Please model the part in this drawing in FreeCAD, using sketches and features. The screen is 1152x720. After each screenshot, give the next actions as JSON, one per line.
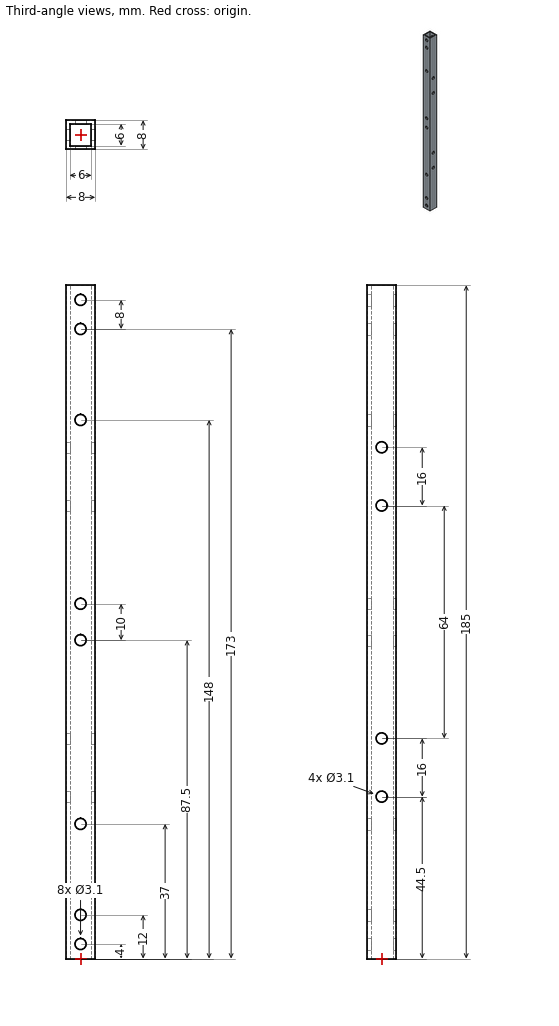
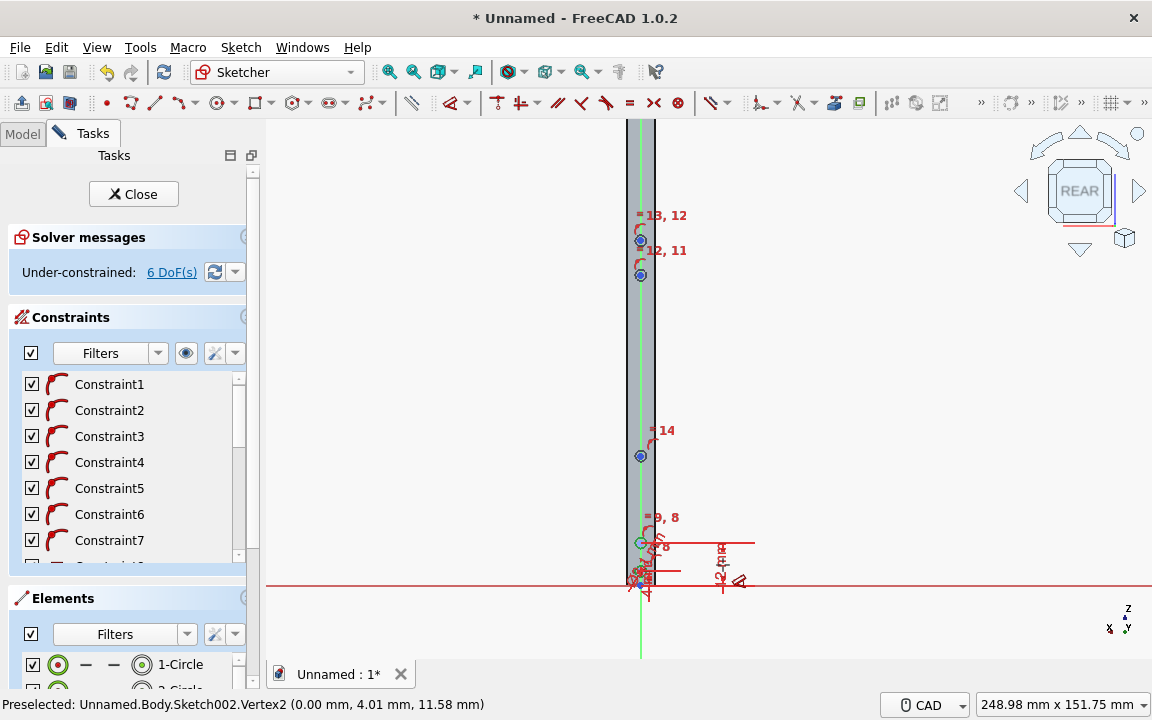
{"action": "left_click", "coordinate": [641, 456]}
{"action": "left_click", "coordinate": [675, 521]}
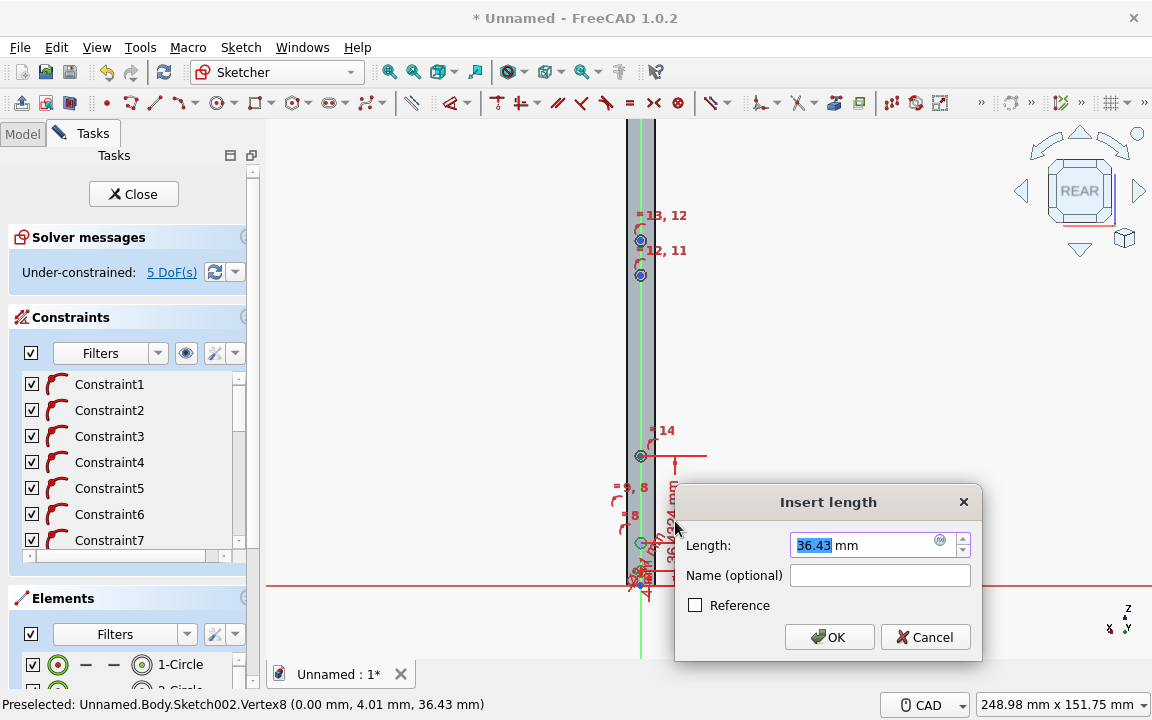
{"action": "type", "text": "37"}
{"action": "key", "text": "Return"}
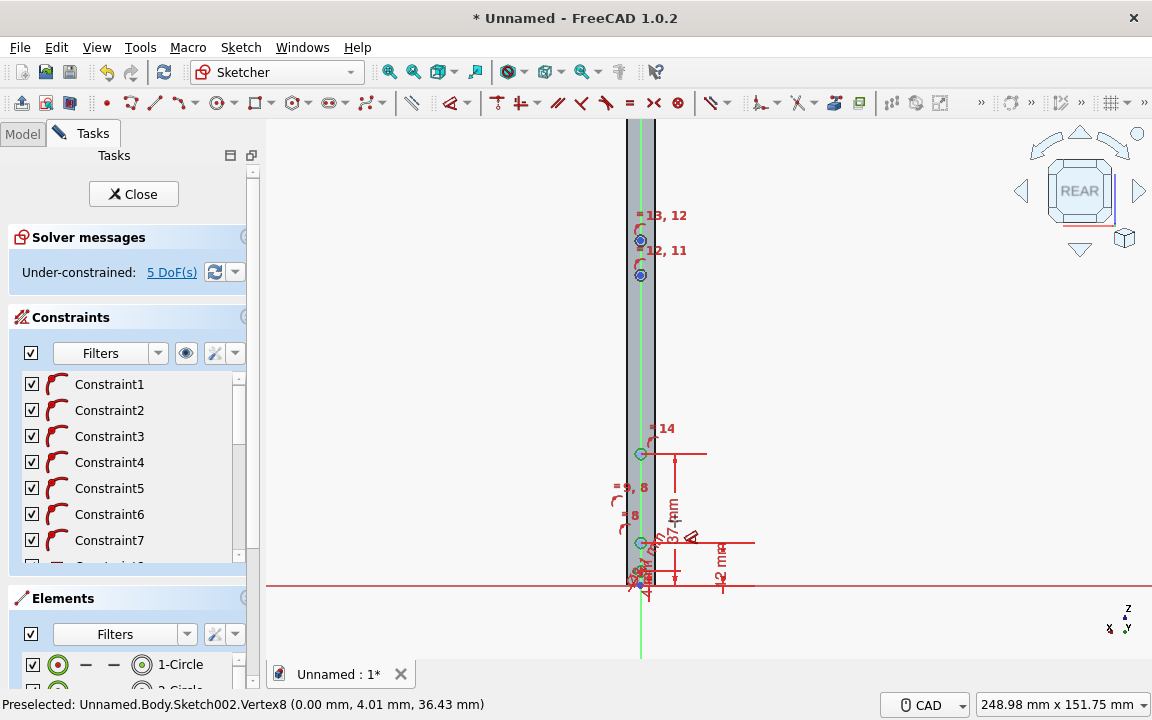
{"action": "scroll", "coordinate": [640, 545], "scroll_direction": "down", "scroll_amount": 3}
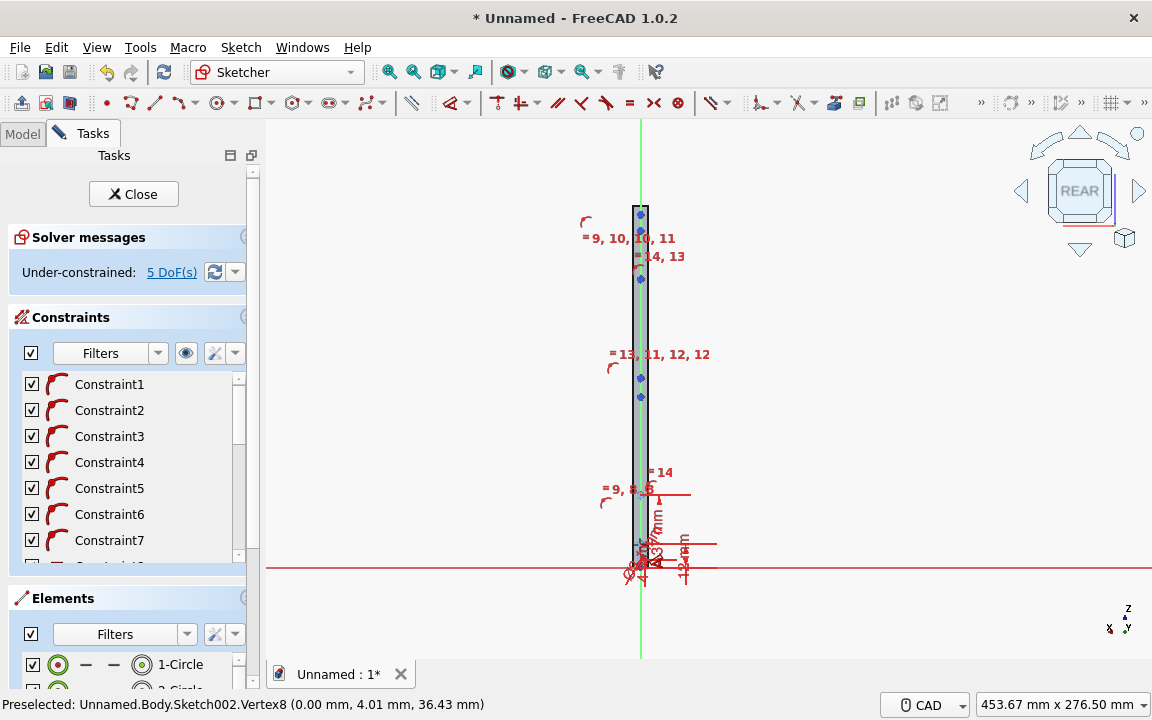
{"action": "scroll", "coordinate": [641, 231], "scroll_direction": "up", "scroll_amount": 5}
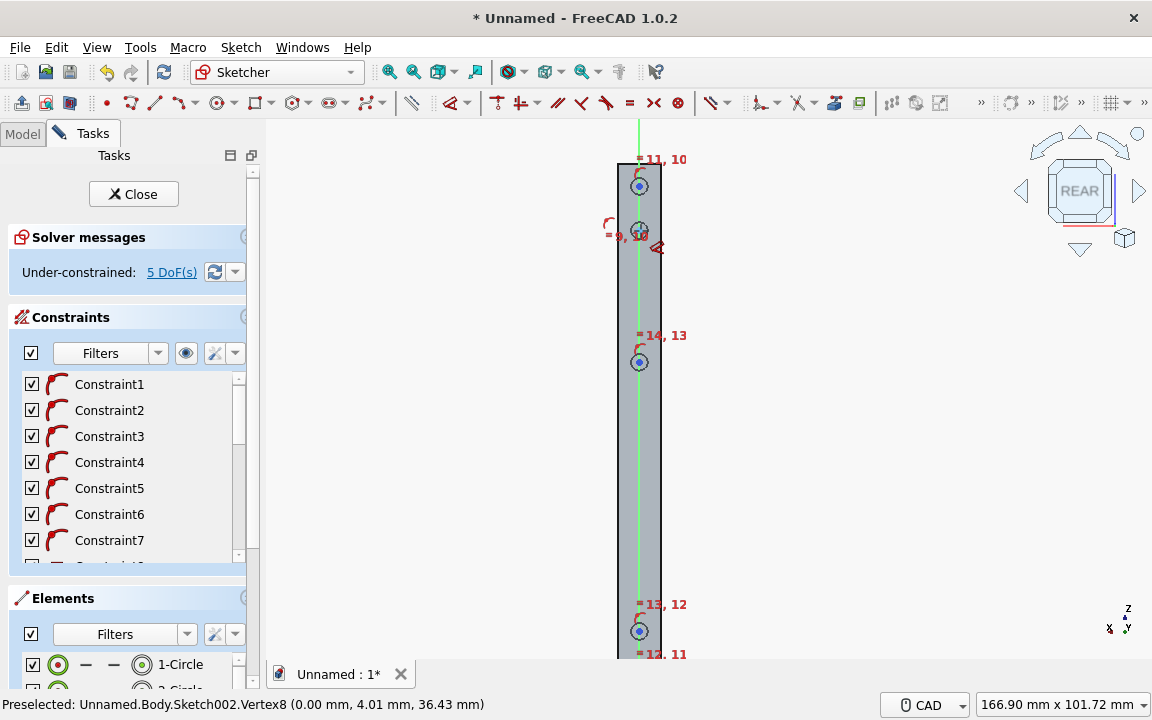
{"action": "left_click", "coordinate": [639, 231]}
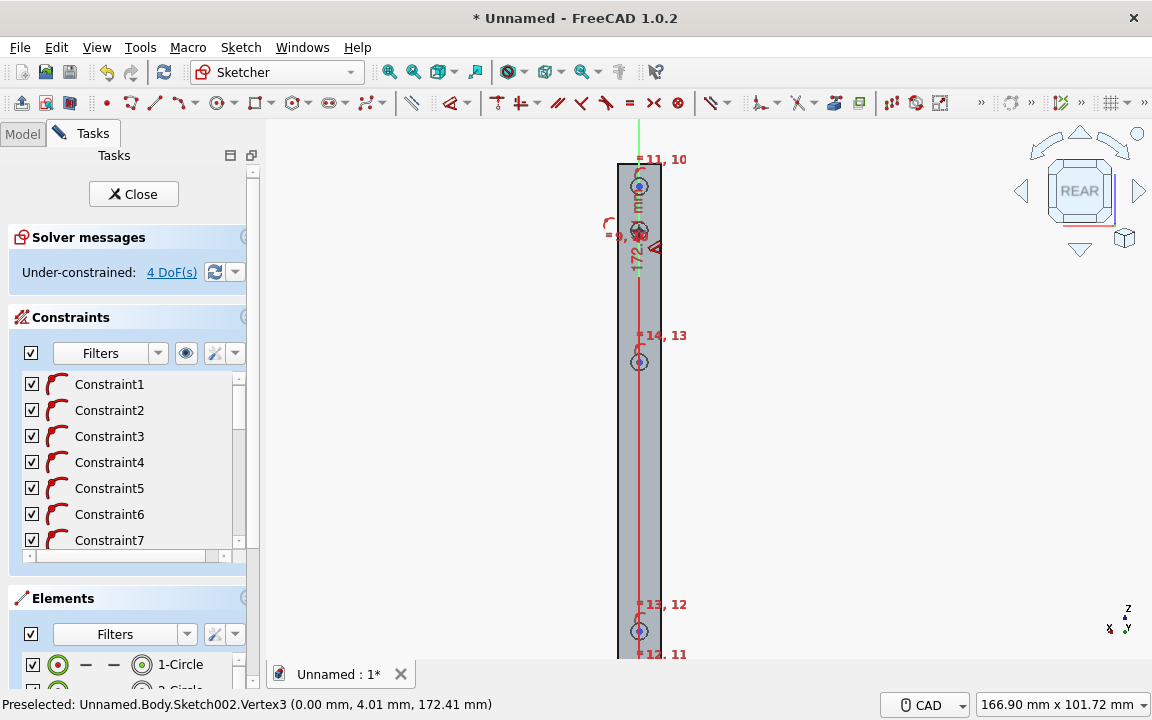
{"action": "left_click", "coordinate": [639, 186]}
{"action": "left_click", "coordinate": [673, 208]}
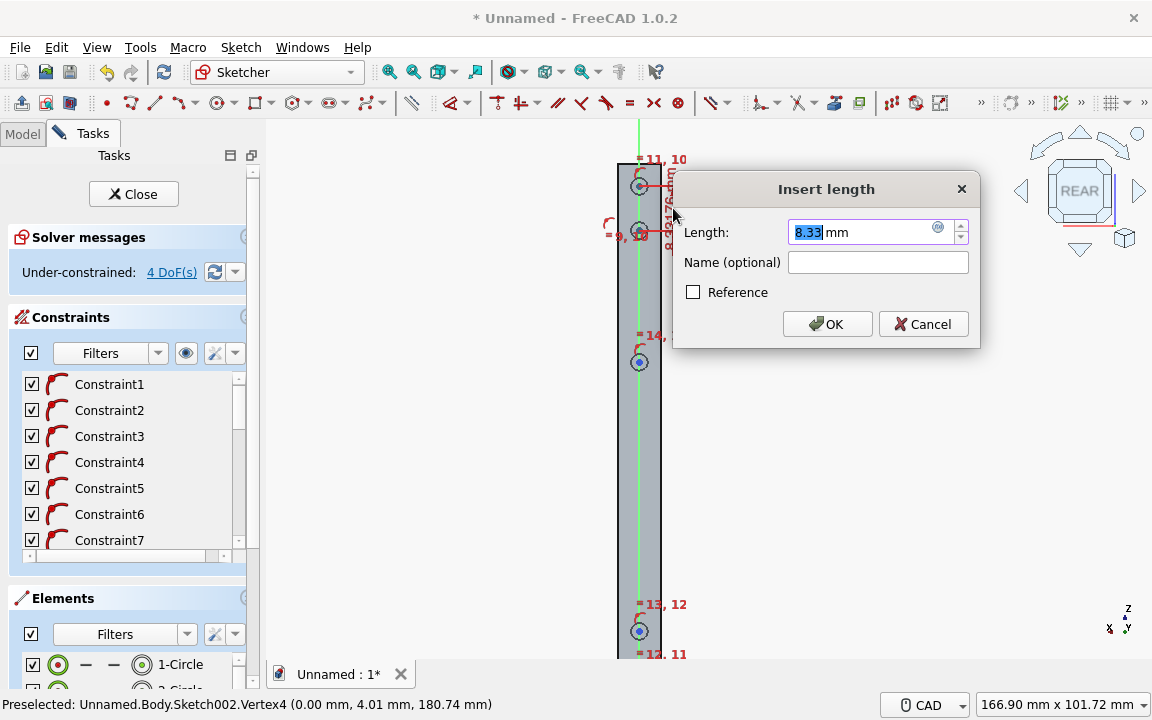
{"action": "type", "text": "8"}
{"action": "key", "text": "Return"}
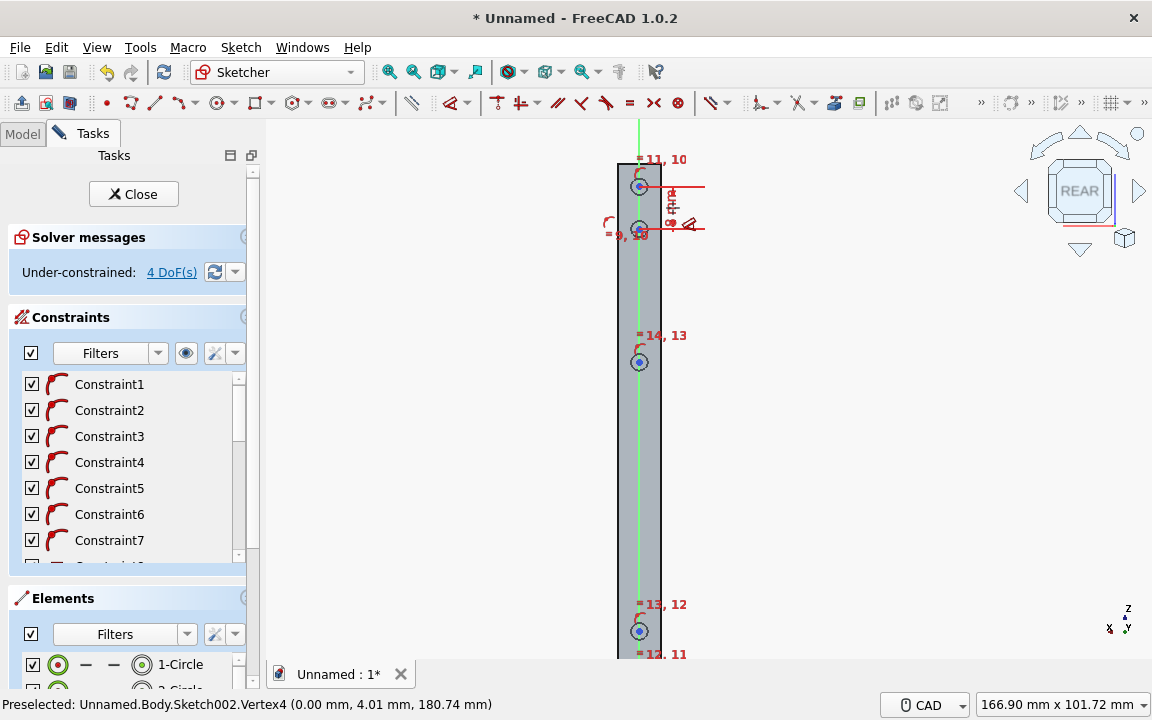
{"action": "left_click", "coordinate": [639, 229]}
{"action": "left_click", "coordinate": [673, 430]}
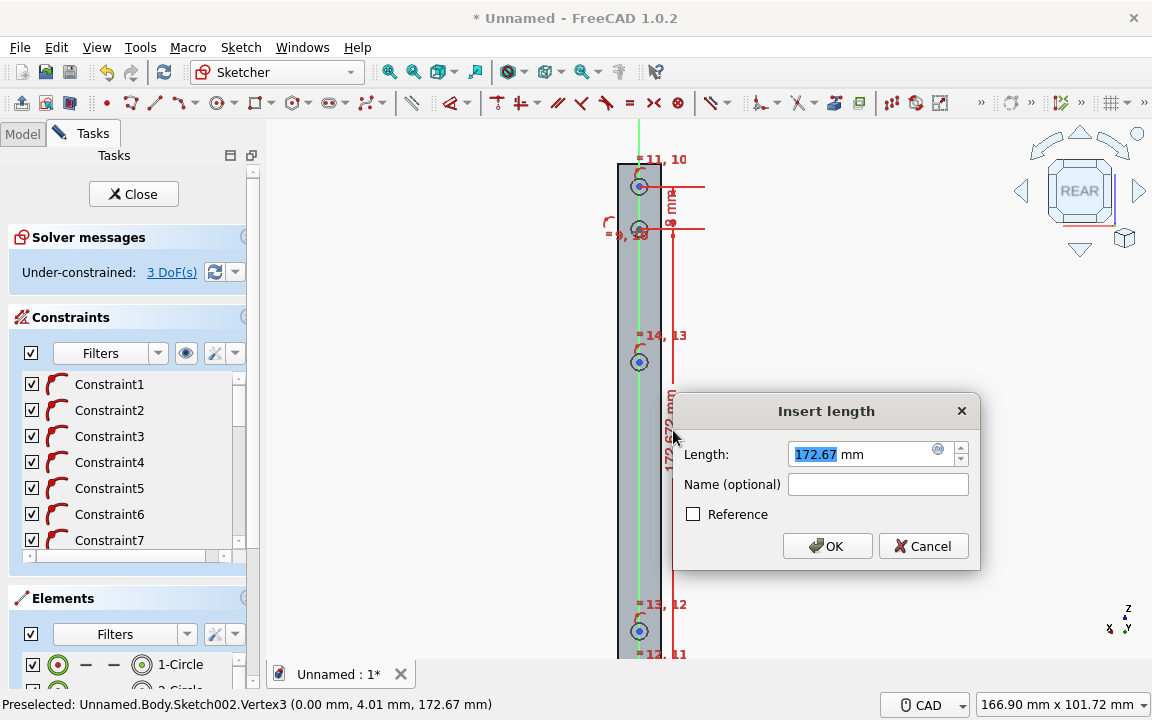
{"action": "type", "text": "173"}
{"action": "key", "text": "Return"}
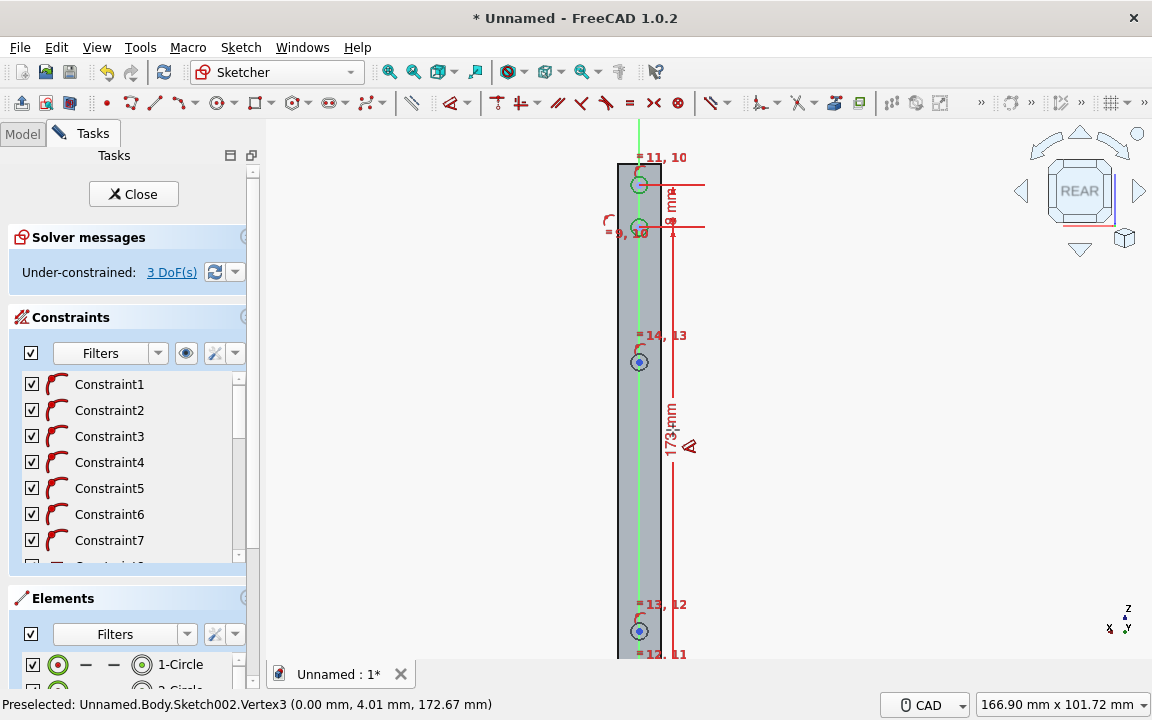
{"action": "left_click", "coordinate": [639, 362]}
{"action": "left_click", "coordinate": [673, 497]}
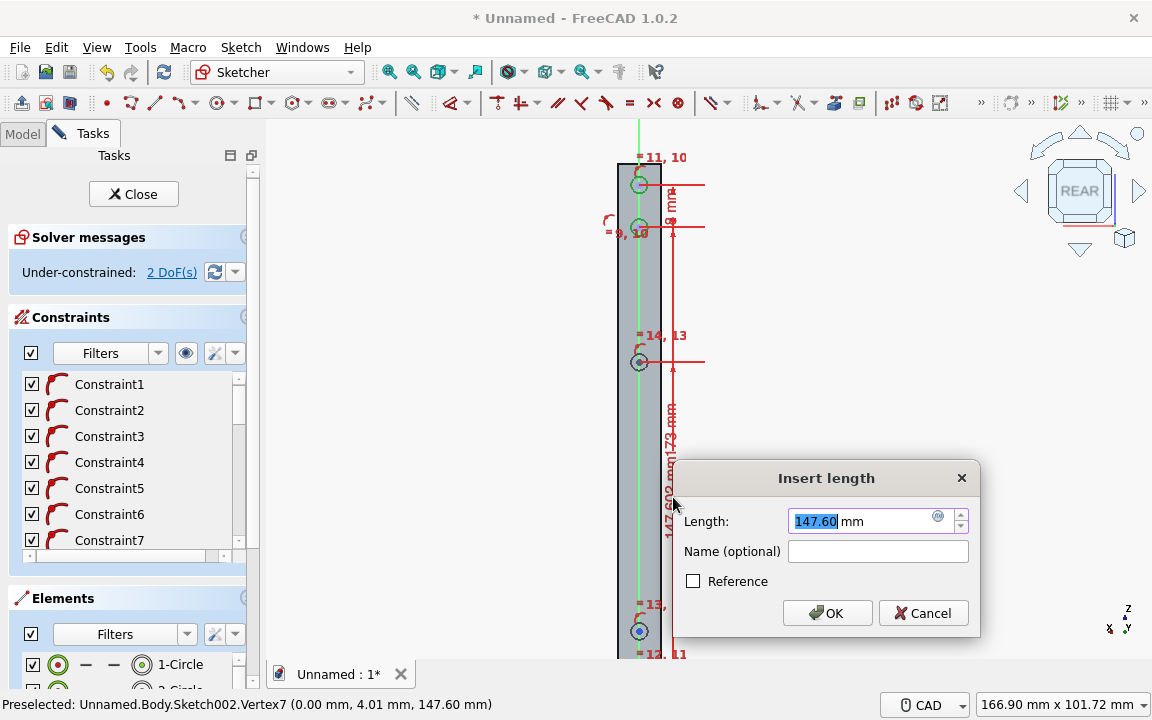
{"action": "type", "text": "148"}
{"action": "key", "text": "Return"}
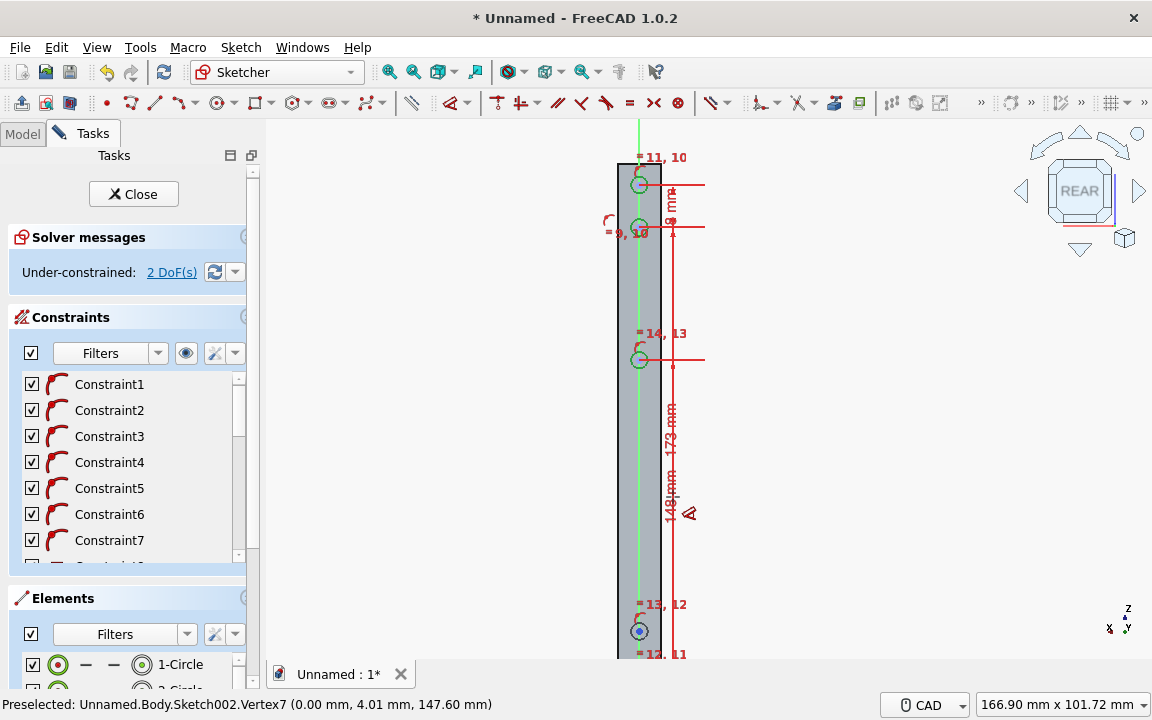
{"action": "scroll", "coordinate": [641, 231], "scroll_direction": "down", "scroll_amount": 5}